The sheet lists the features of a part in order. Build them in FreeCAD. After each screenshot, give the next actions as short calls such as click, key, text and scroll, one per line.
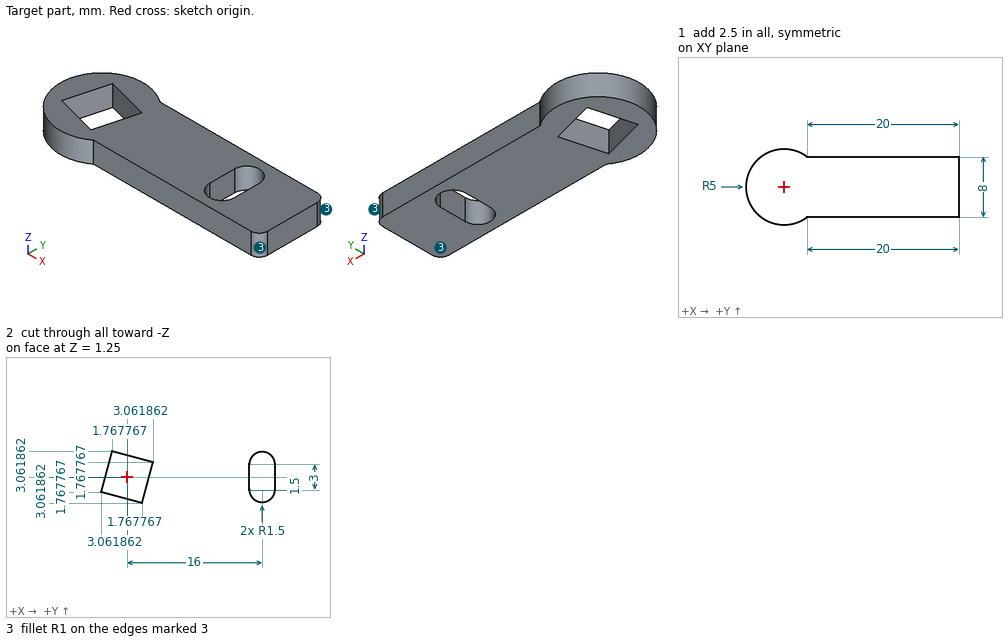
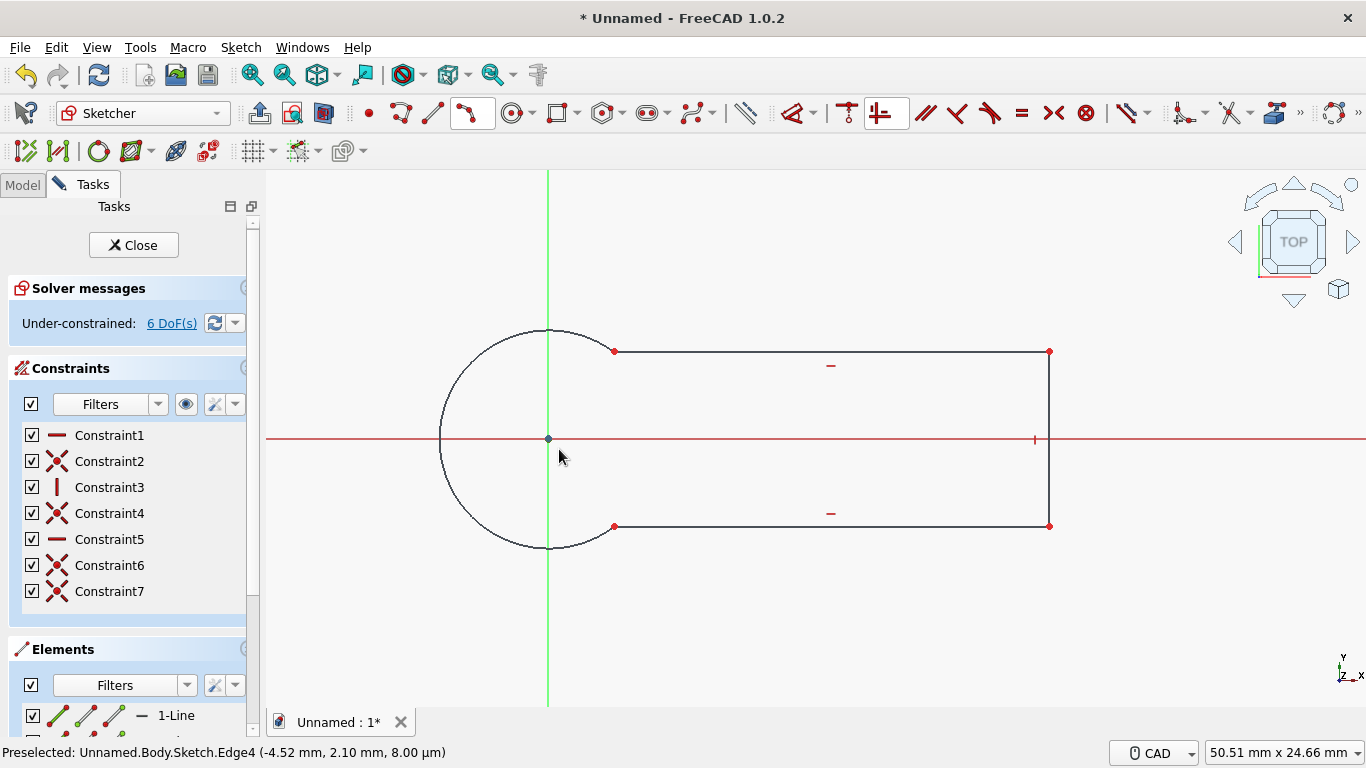
click(848, 114)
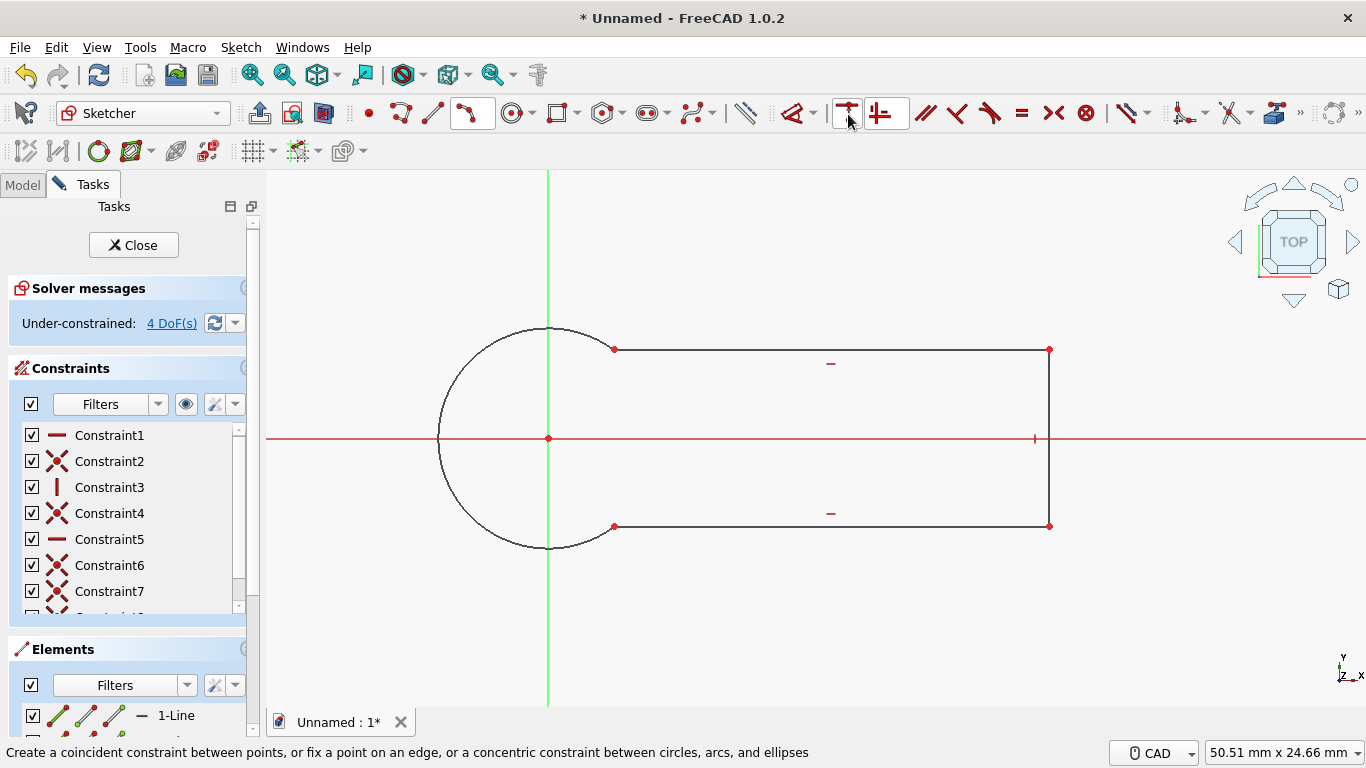
key(d)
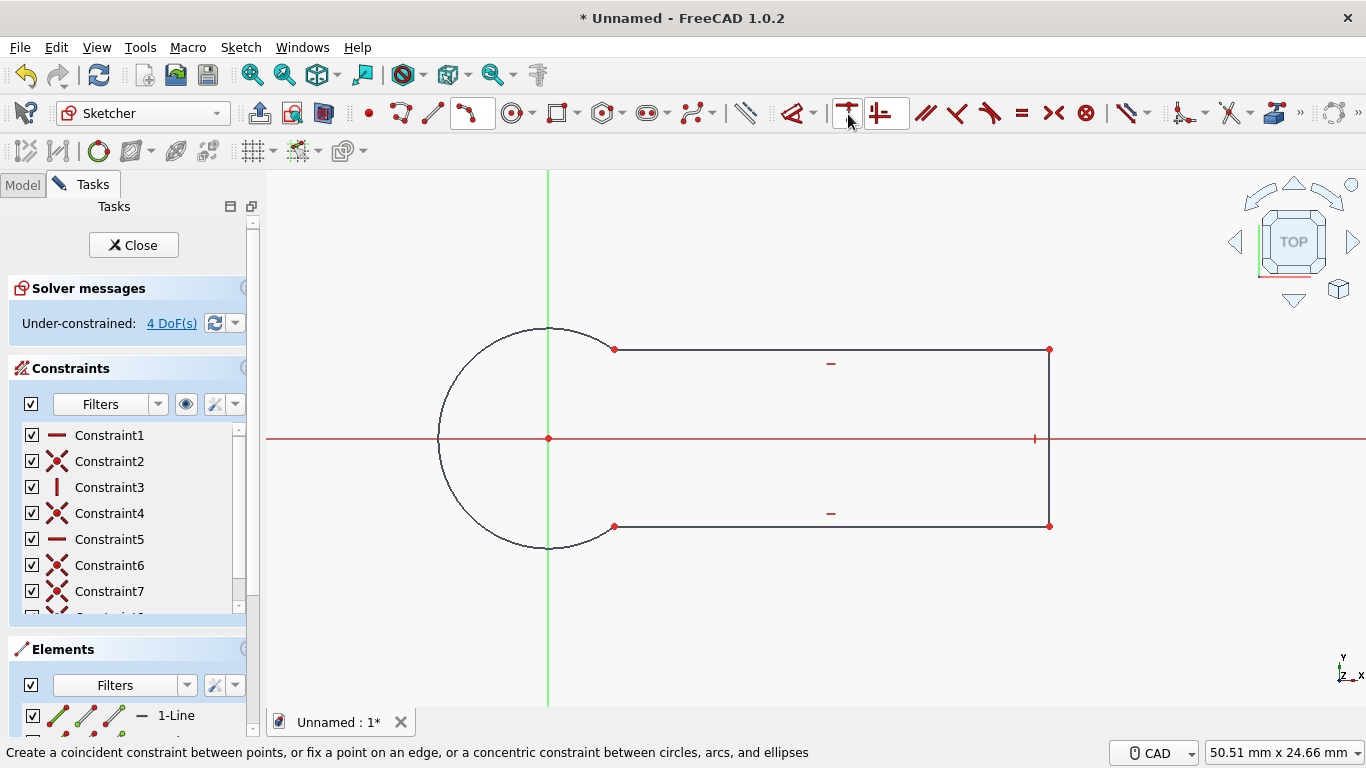
click(479, 353)
click(459, 328)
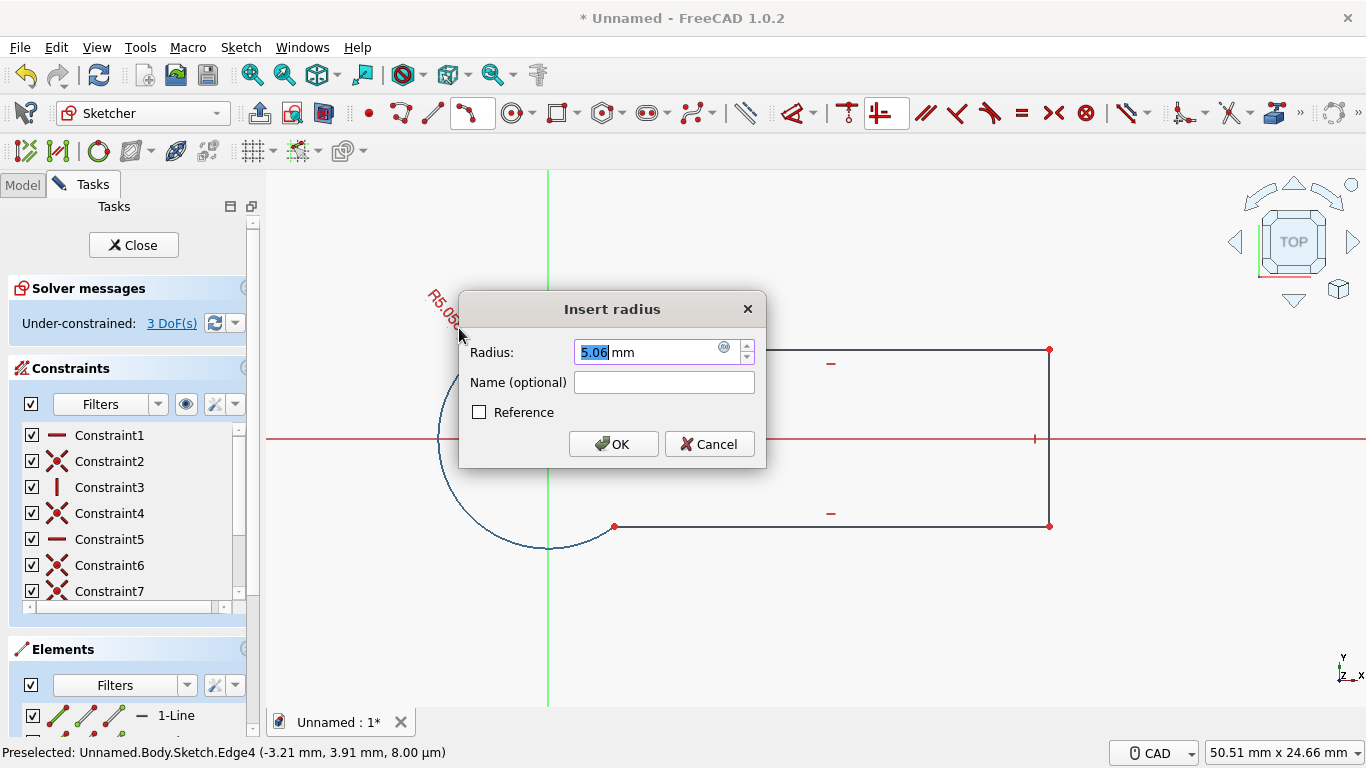
text(5)
key(Return)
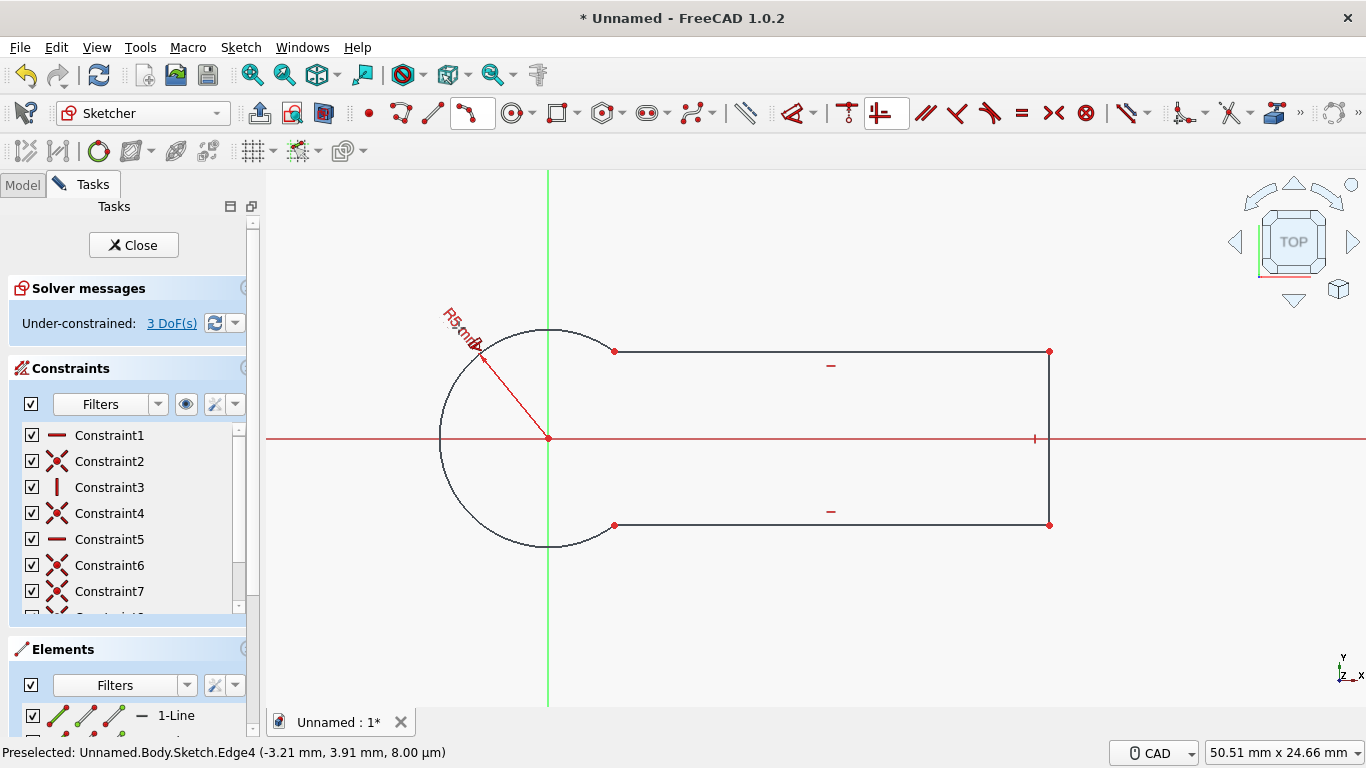
click(1049, 473)
click(1083, 399)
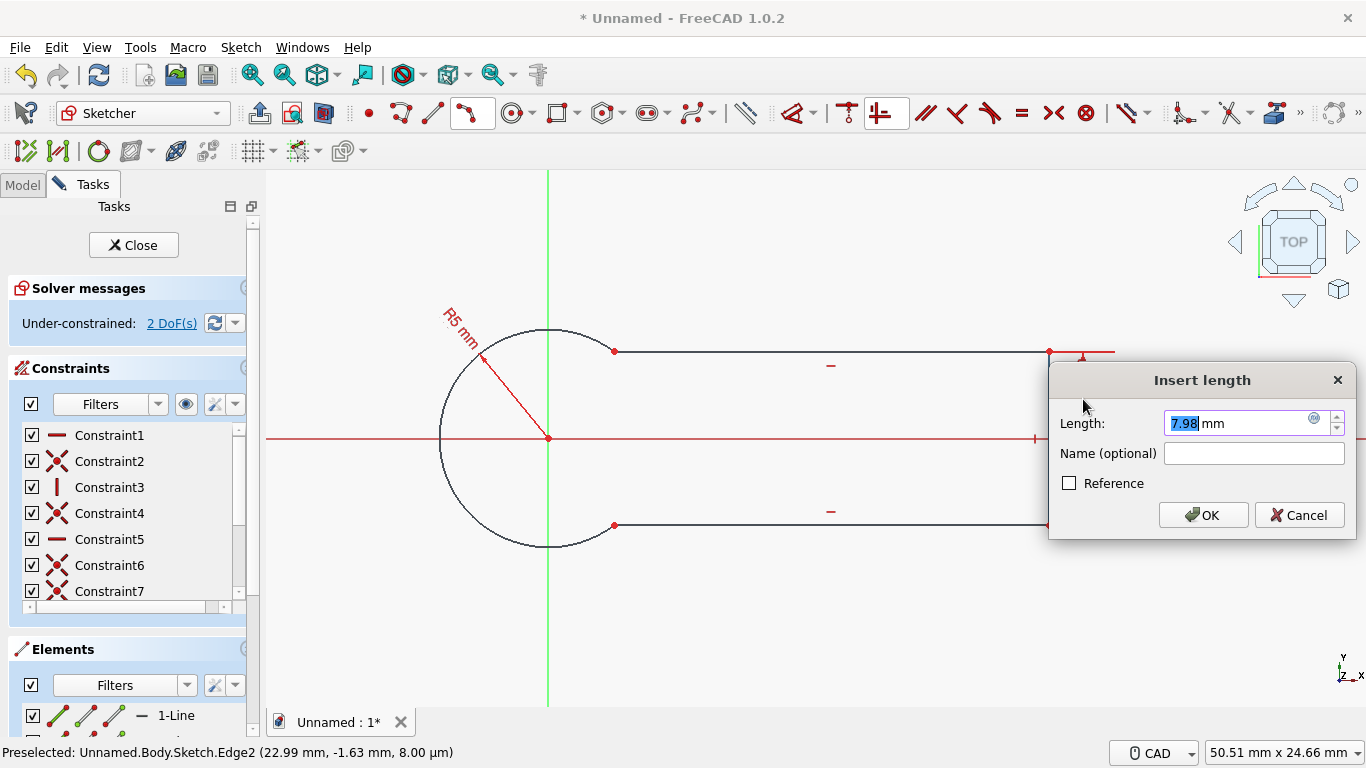
text(8)
key(Return)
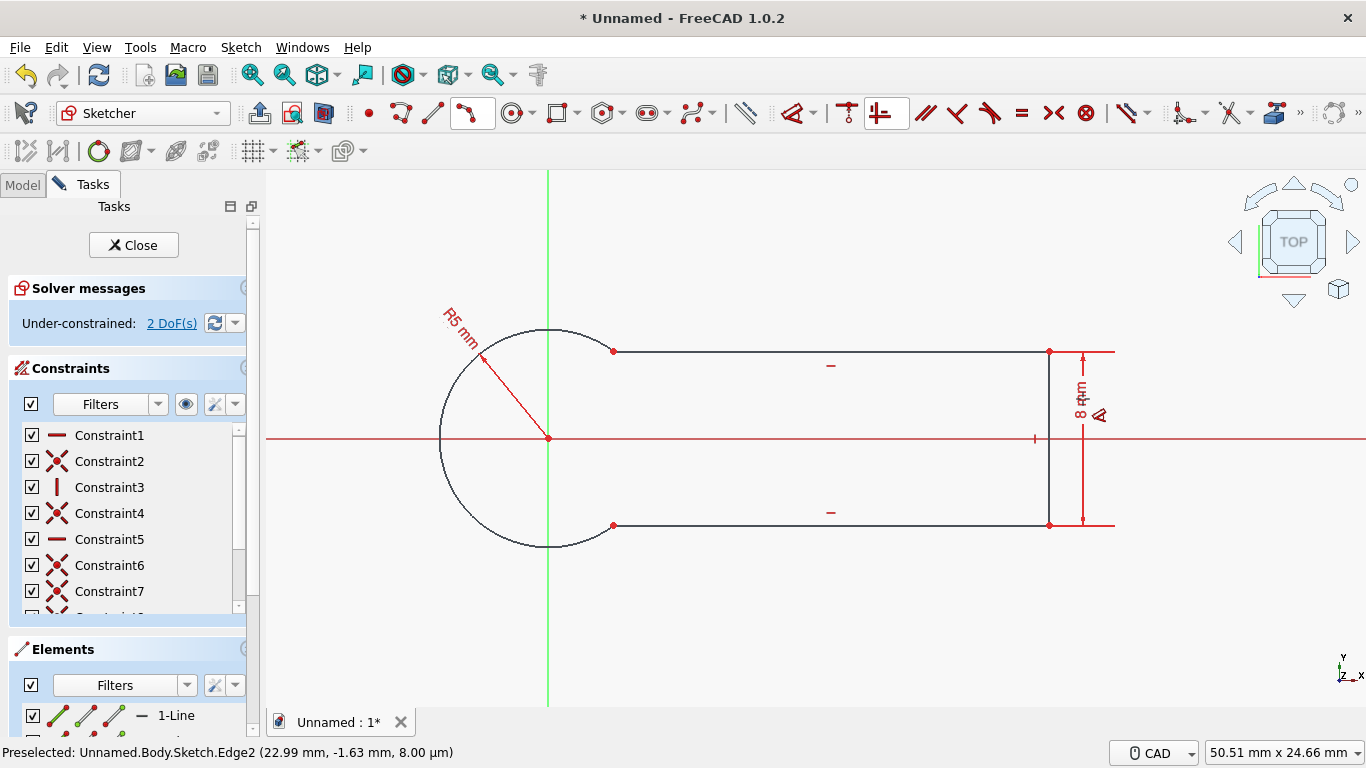
click(744, 526)
click(831, 560)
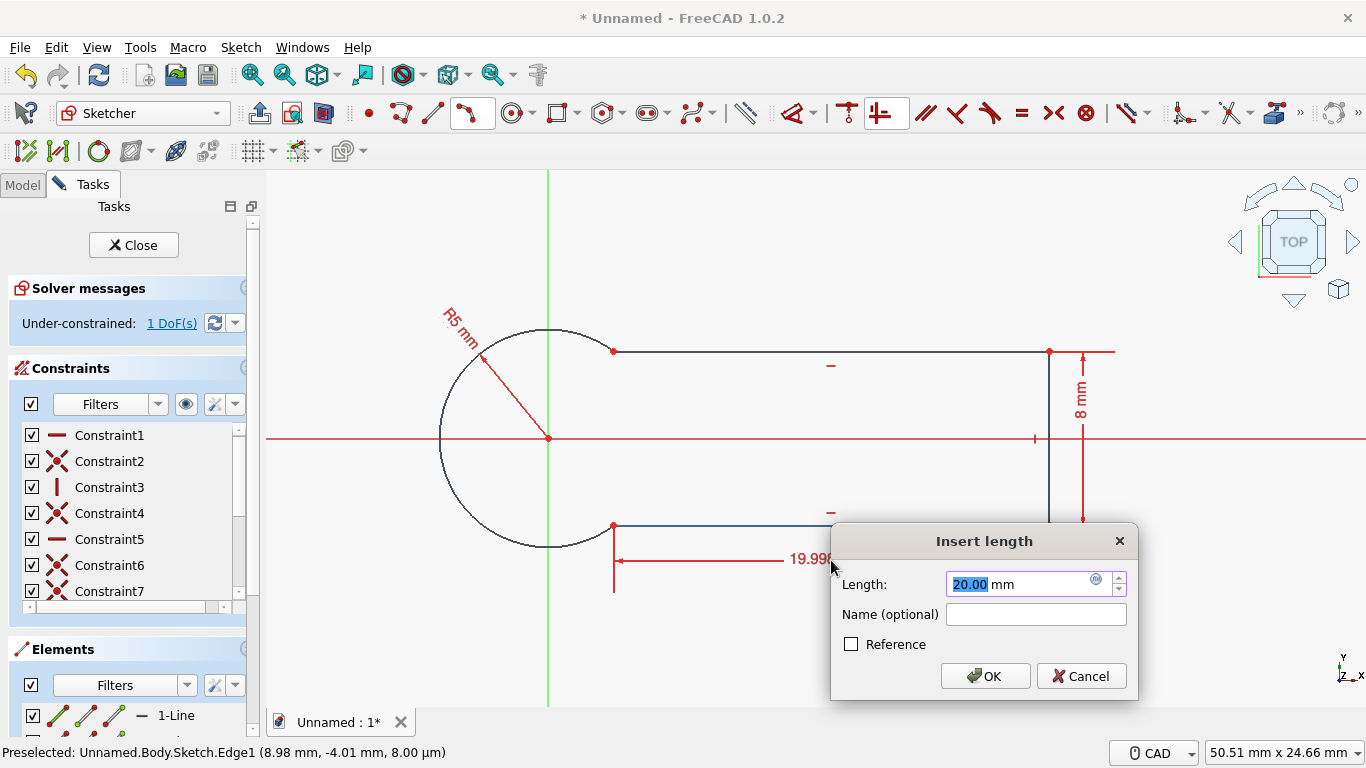
text(20)
key(Return)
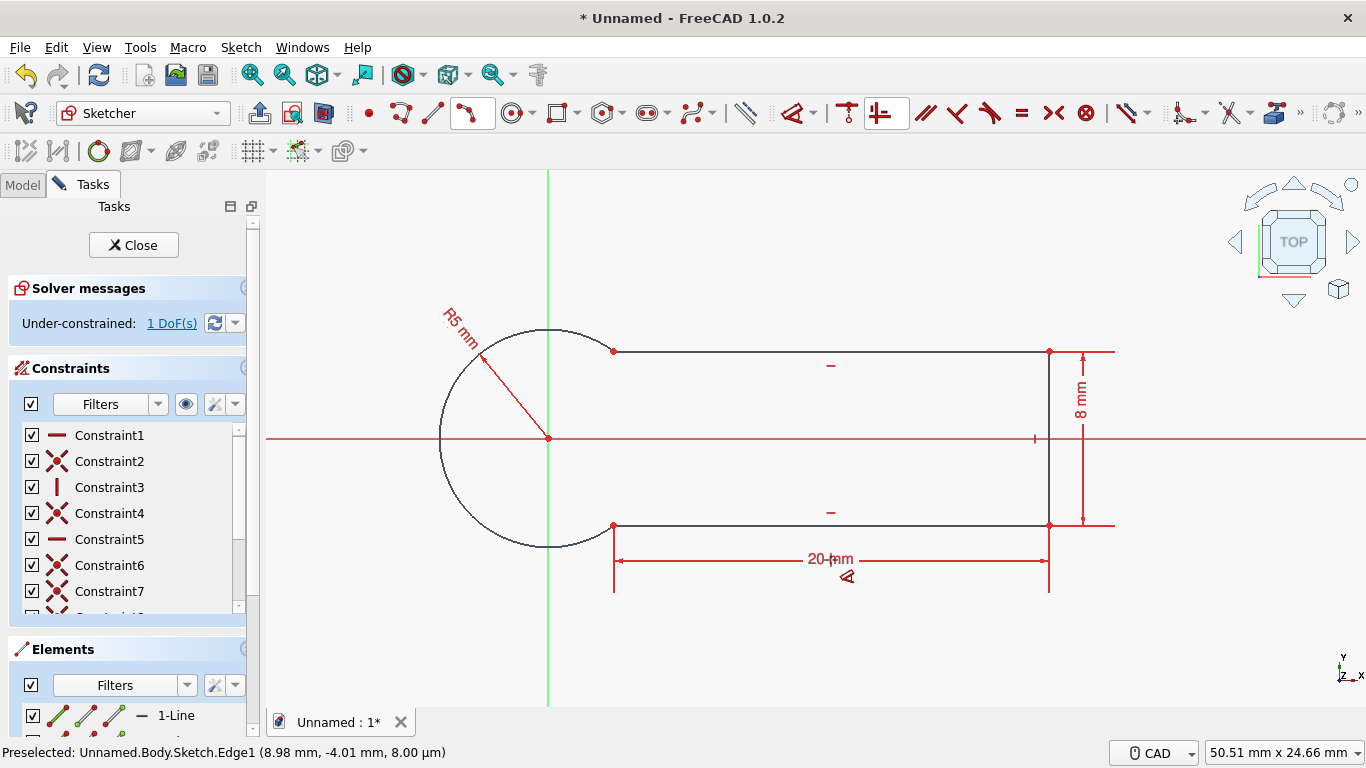
click(919, 352)
click(832, 318)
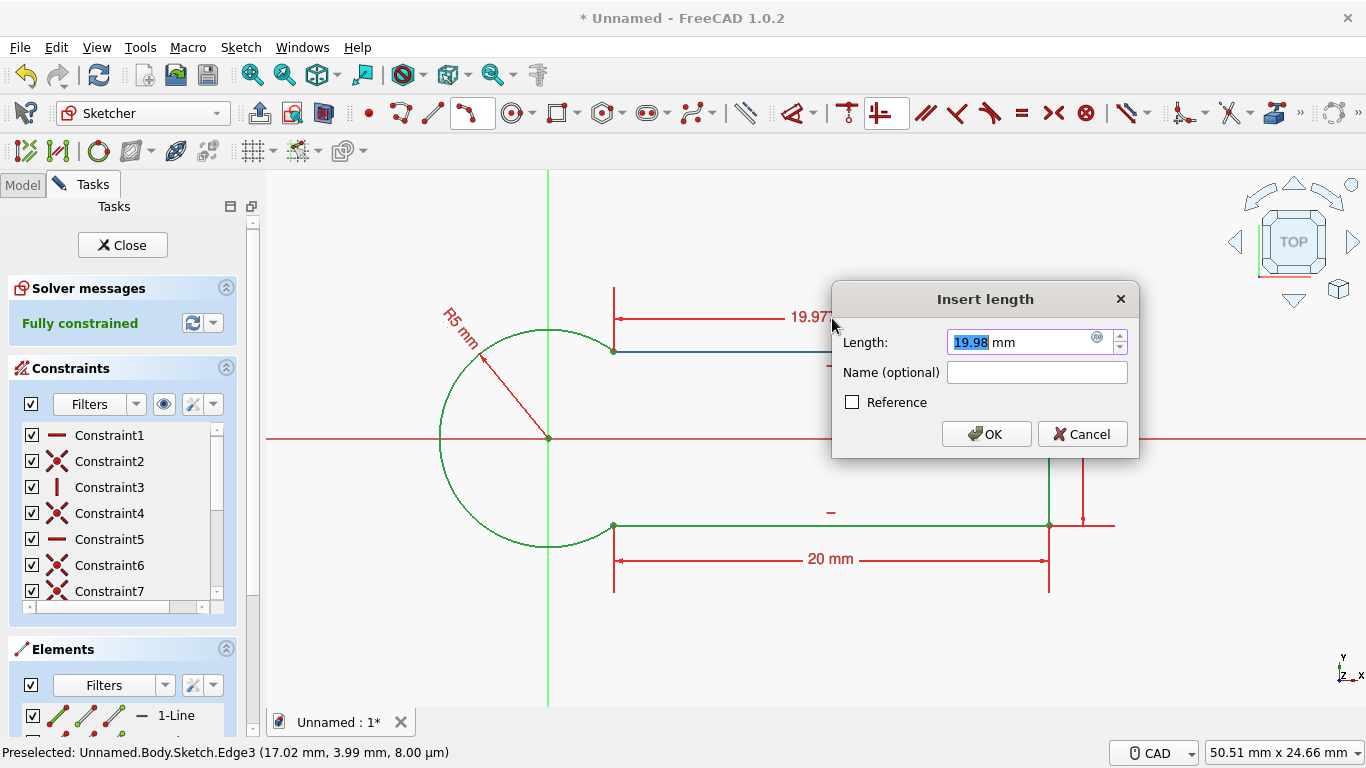
text(20)
key(Return)
key(Escape)